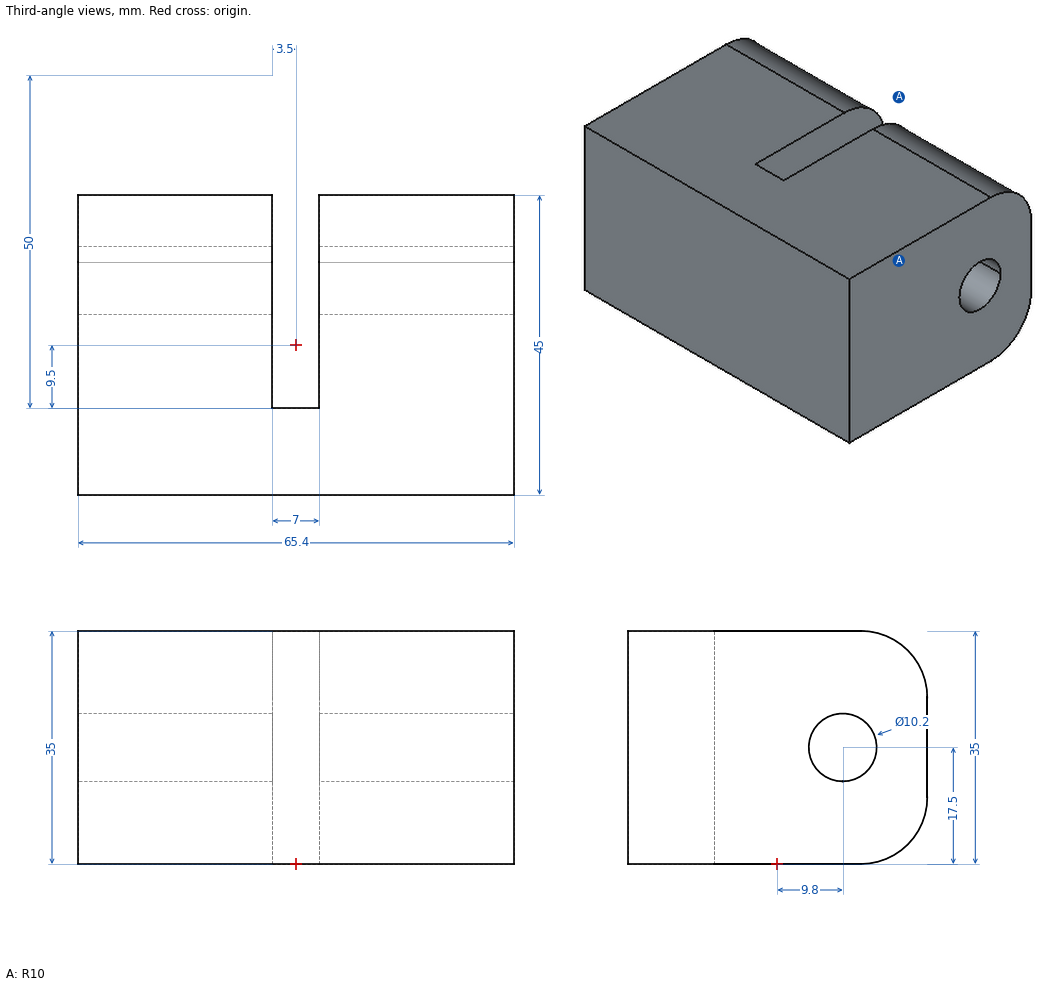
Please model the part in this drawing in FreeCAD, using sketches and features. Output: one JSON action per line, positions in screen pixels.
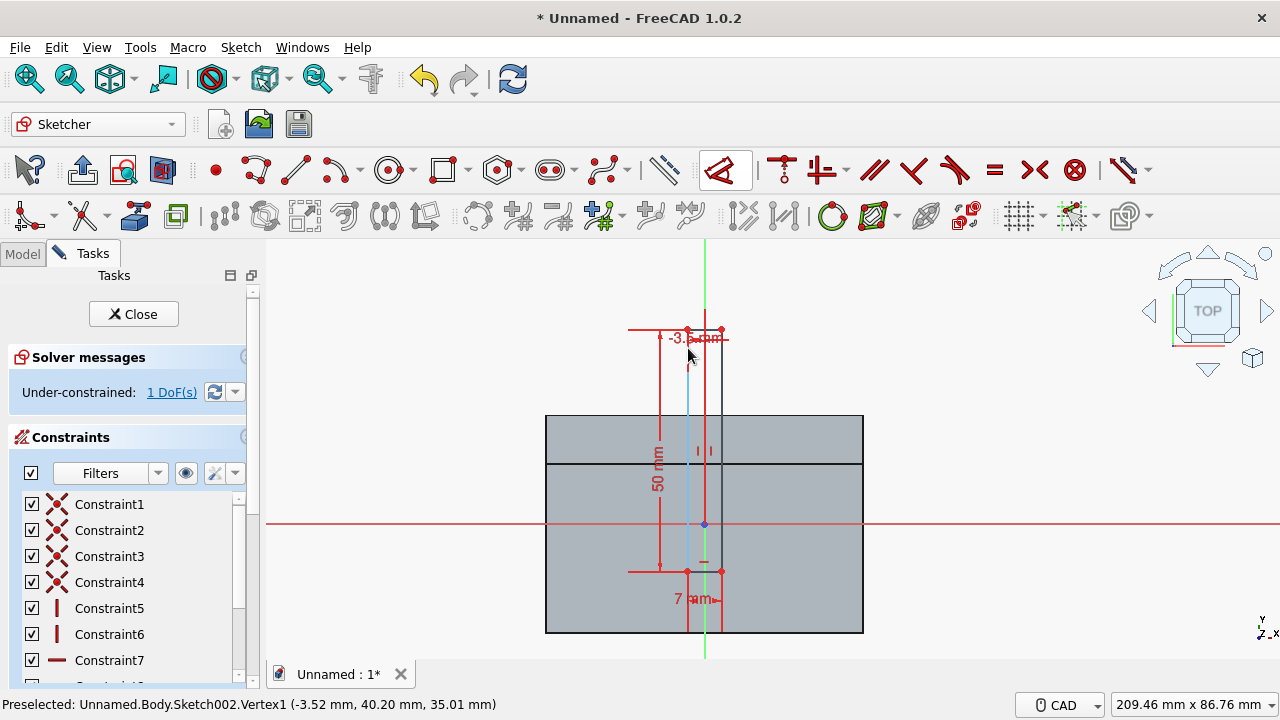
{"action": "left_click", "coordinate": [688, 572]}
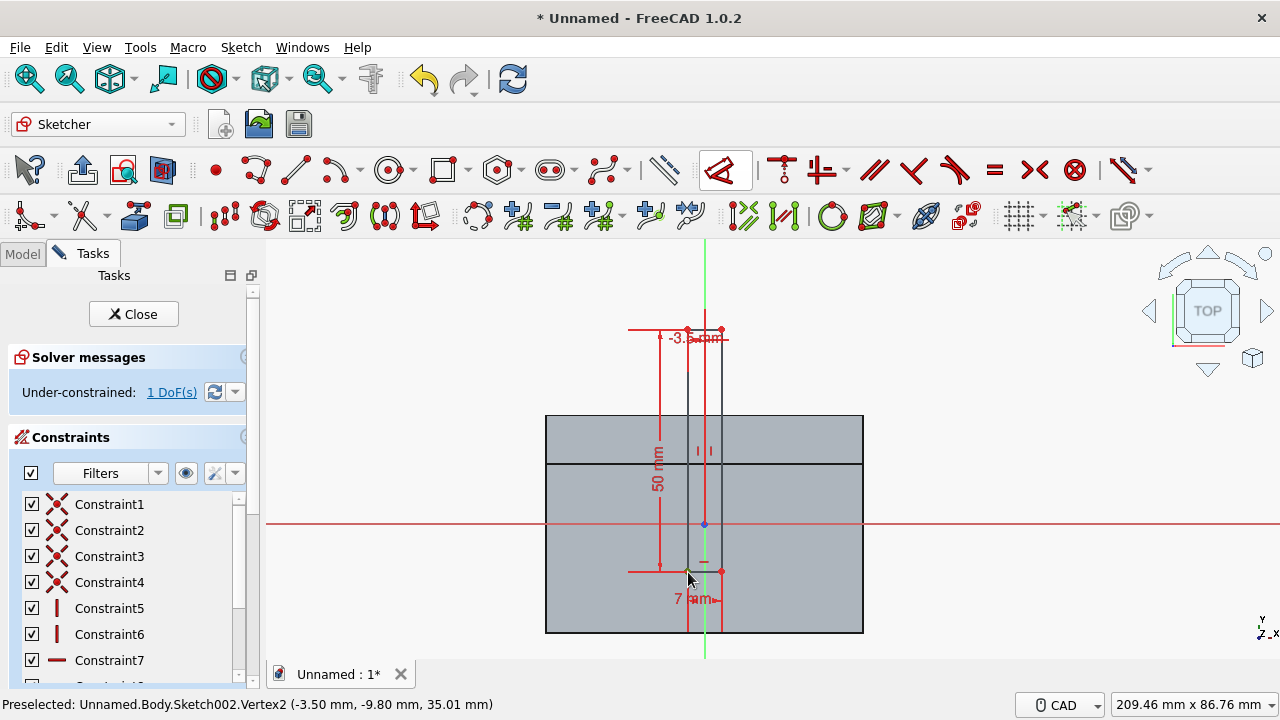
{"action": "left_click", "coordinate": [746, 170]}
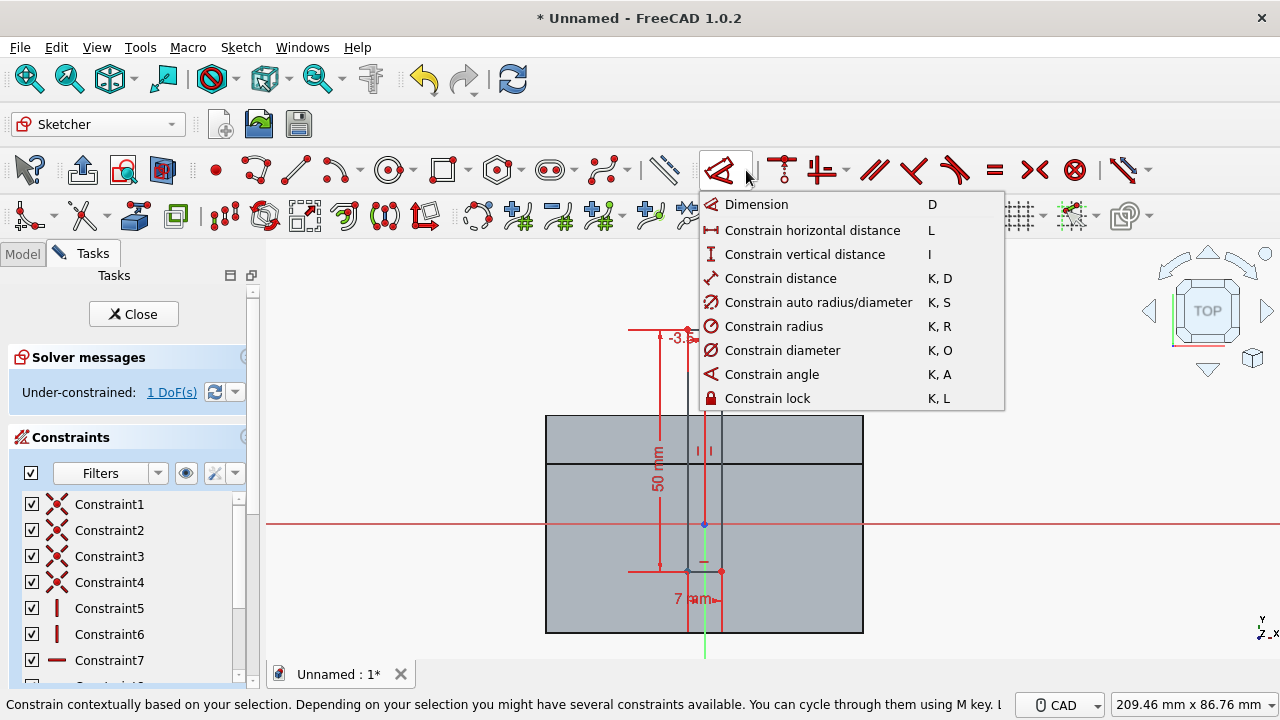
{"action": "left_click", "coordinate": [852, 254]}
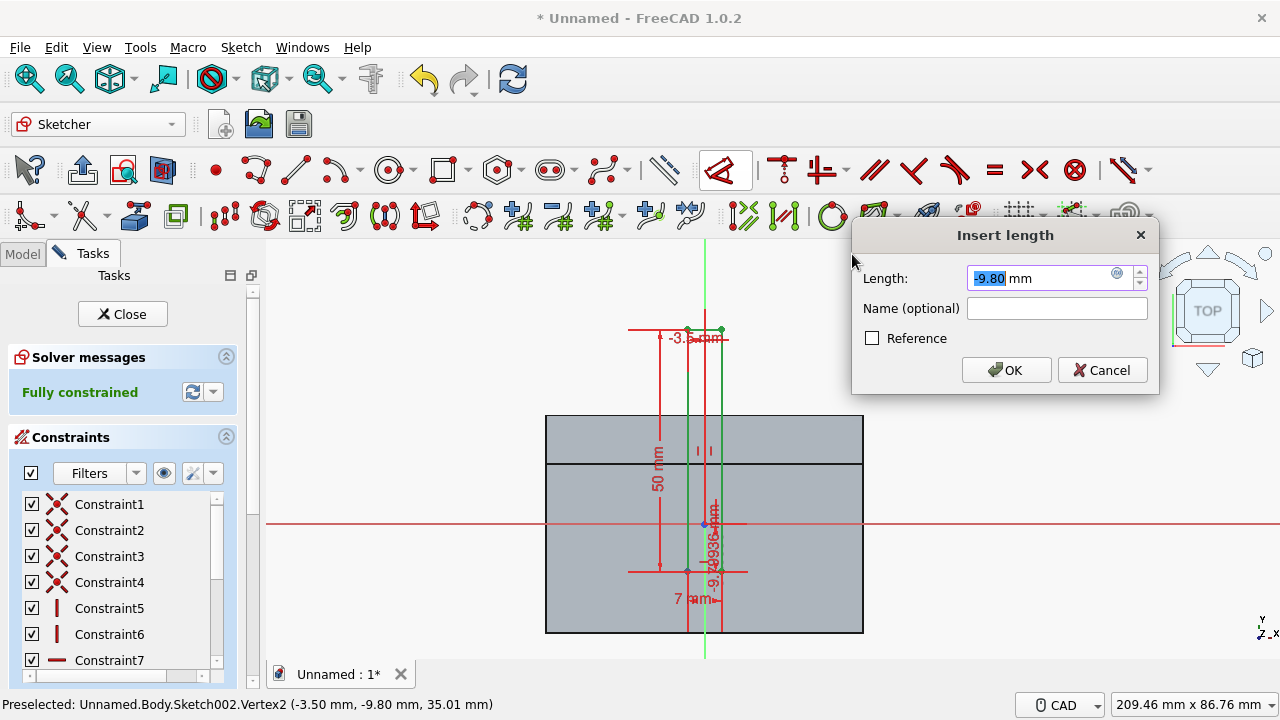
{"action": "type", "text": "-9.5"}
{"action": "key", "text": "Return"}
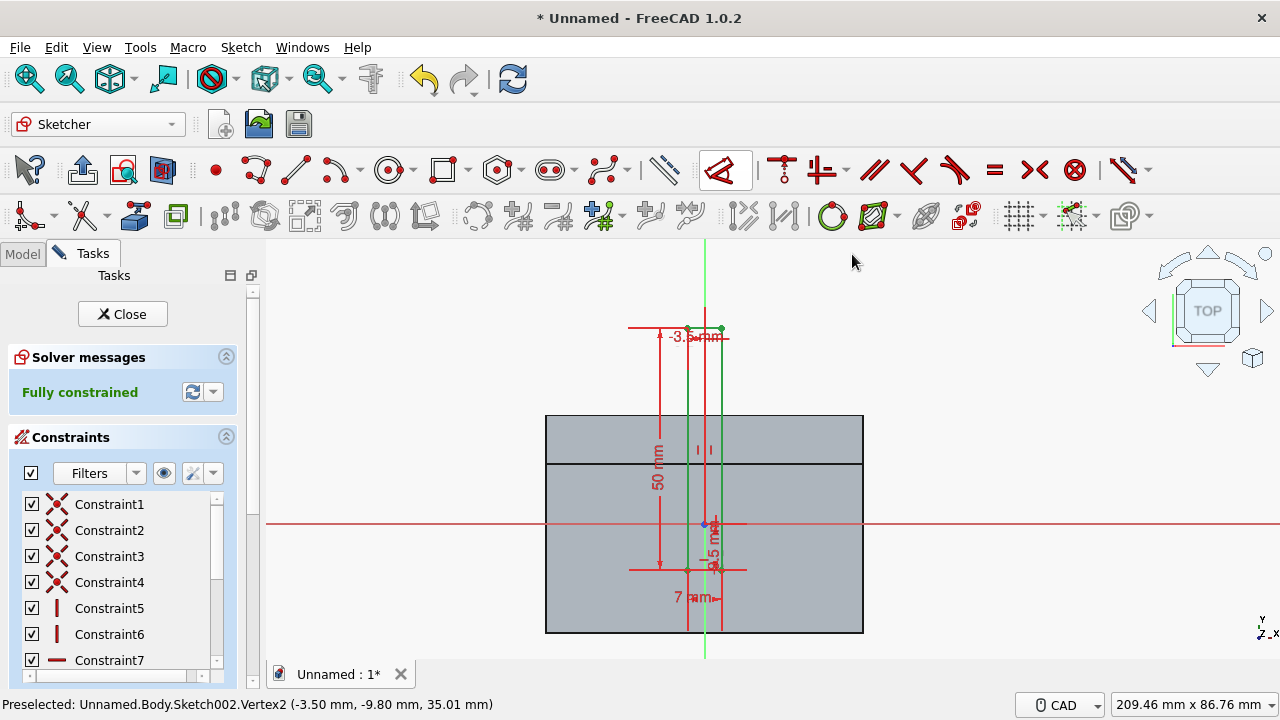
{"action": "left_click", "coordinate": [123, 314]}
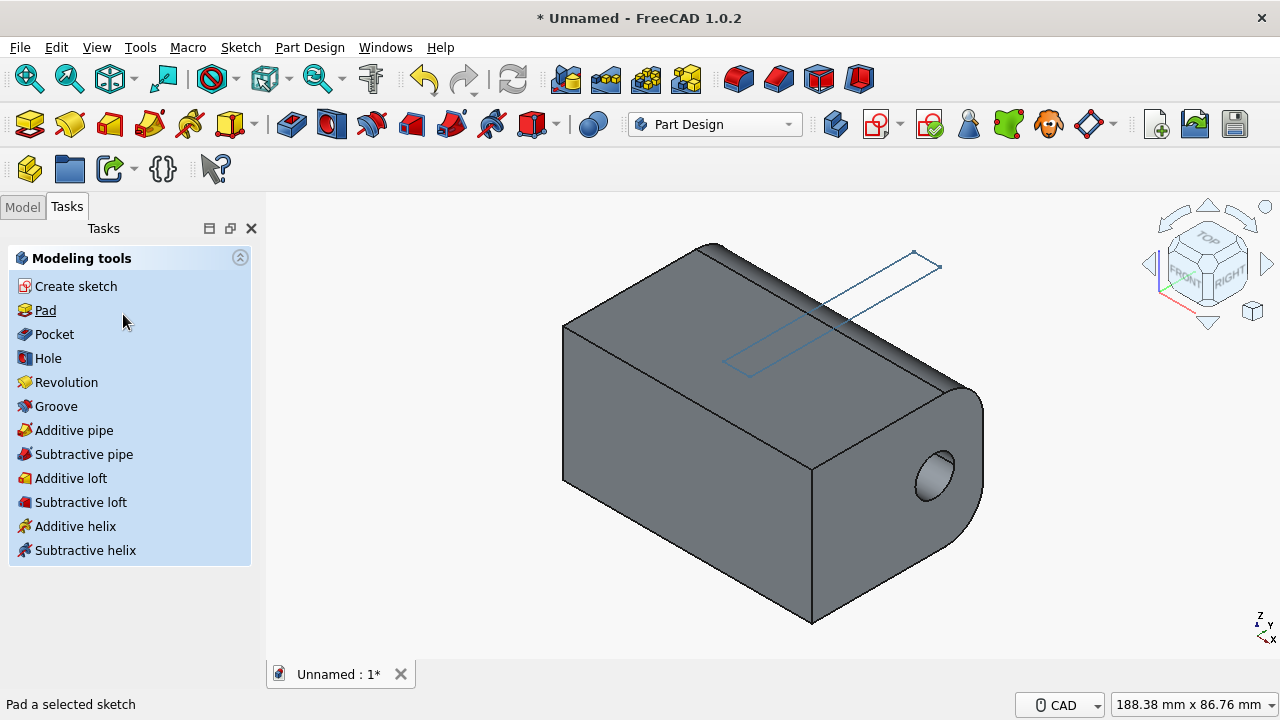
{"action": "left_click", "coordinate": [292, 124]}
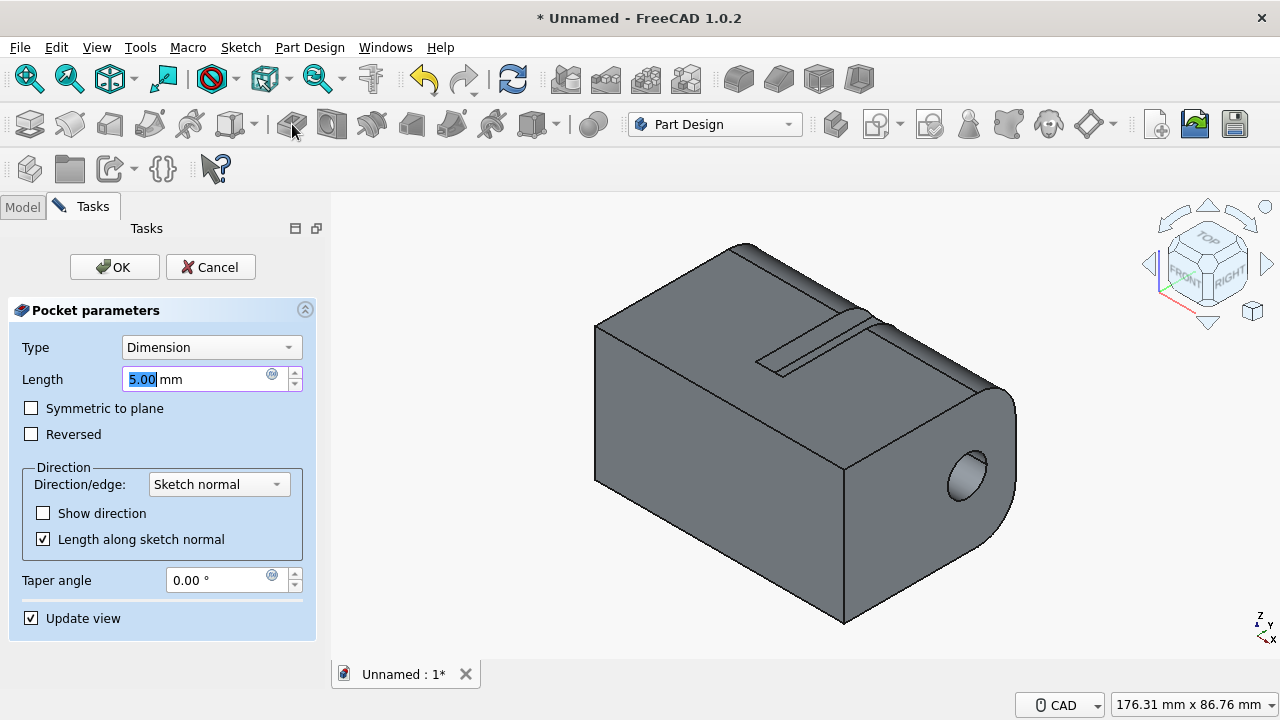
{"action": "type", "text": "35"}
{"action": "key", "text": "Tab"}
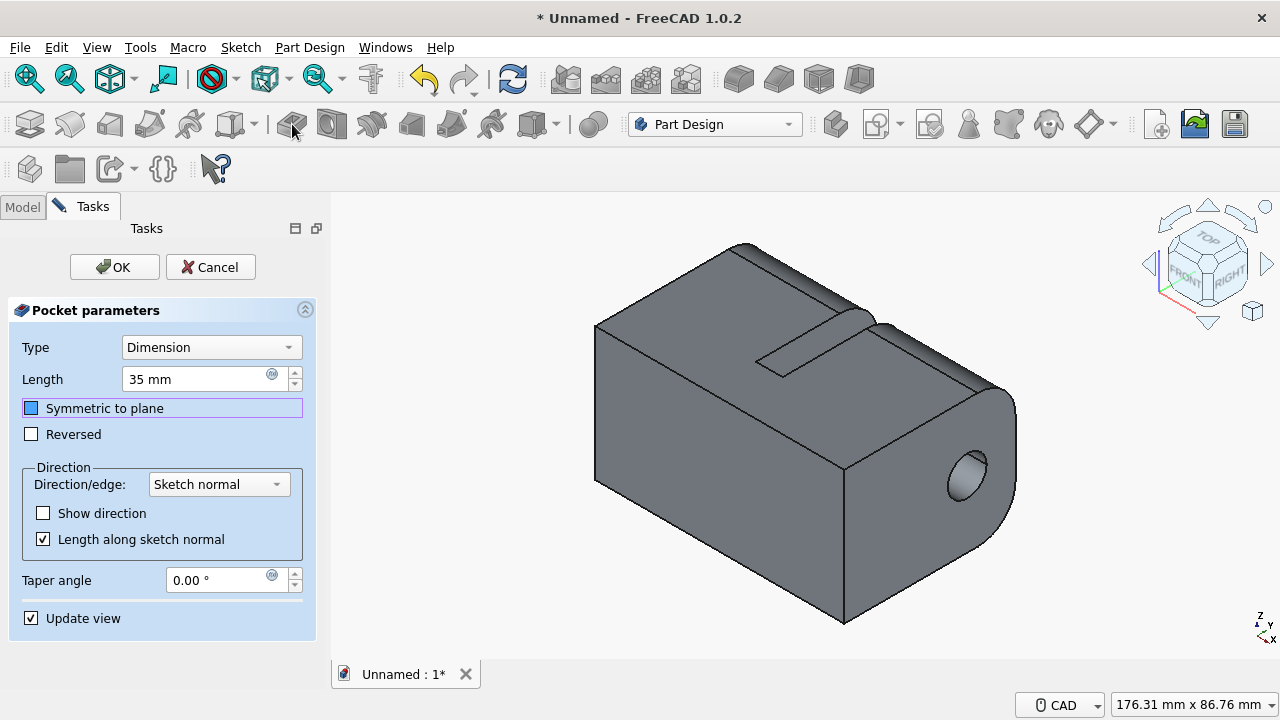
{"action": "left_click", "coordinate": [115, 267]}